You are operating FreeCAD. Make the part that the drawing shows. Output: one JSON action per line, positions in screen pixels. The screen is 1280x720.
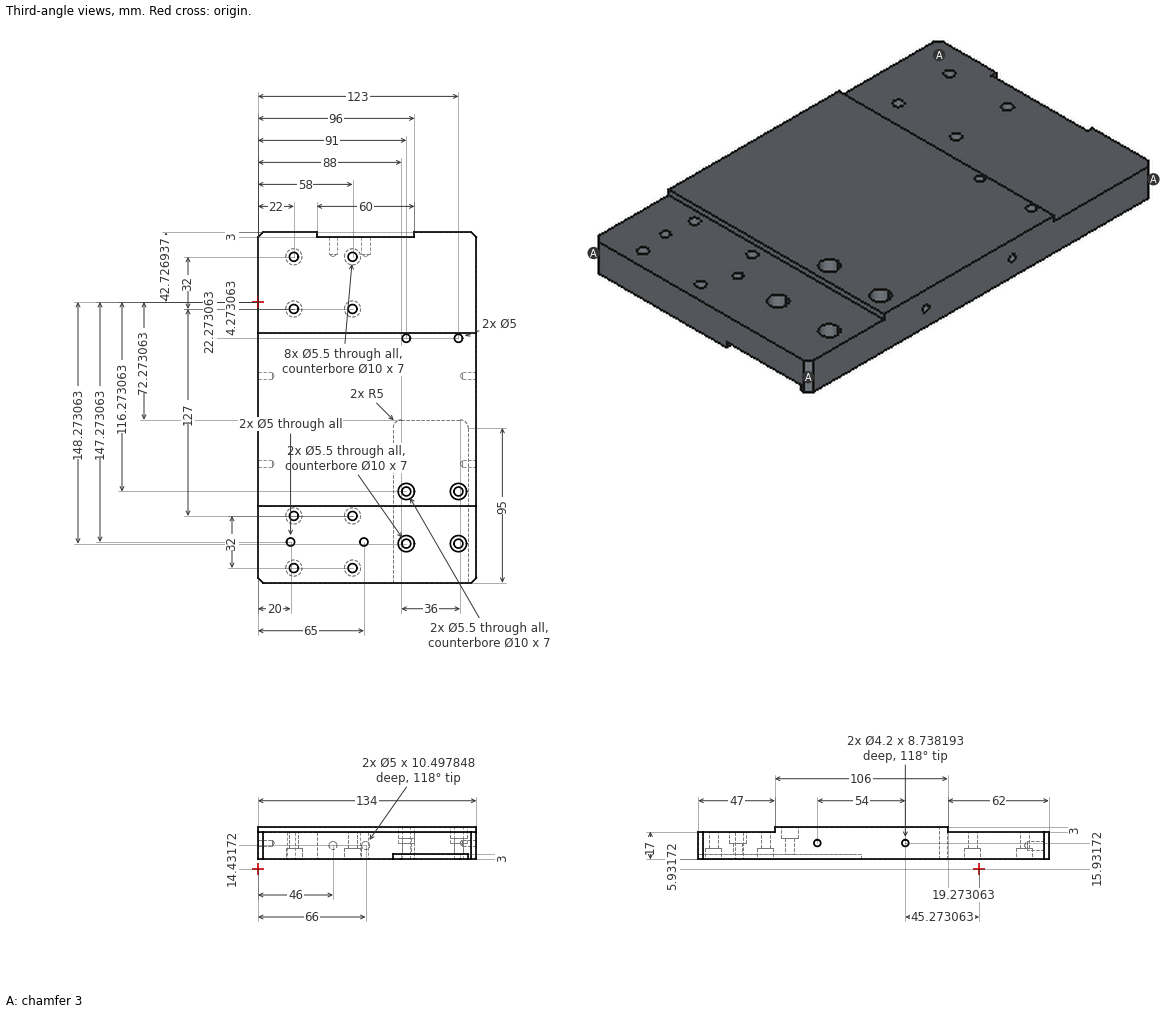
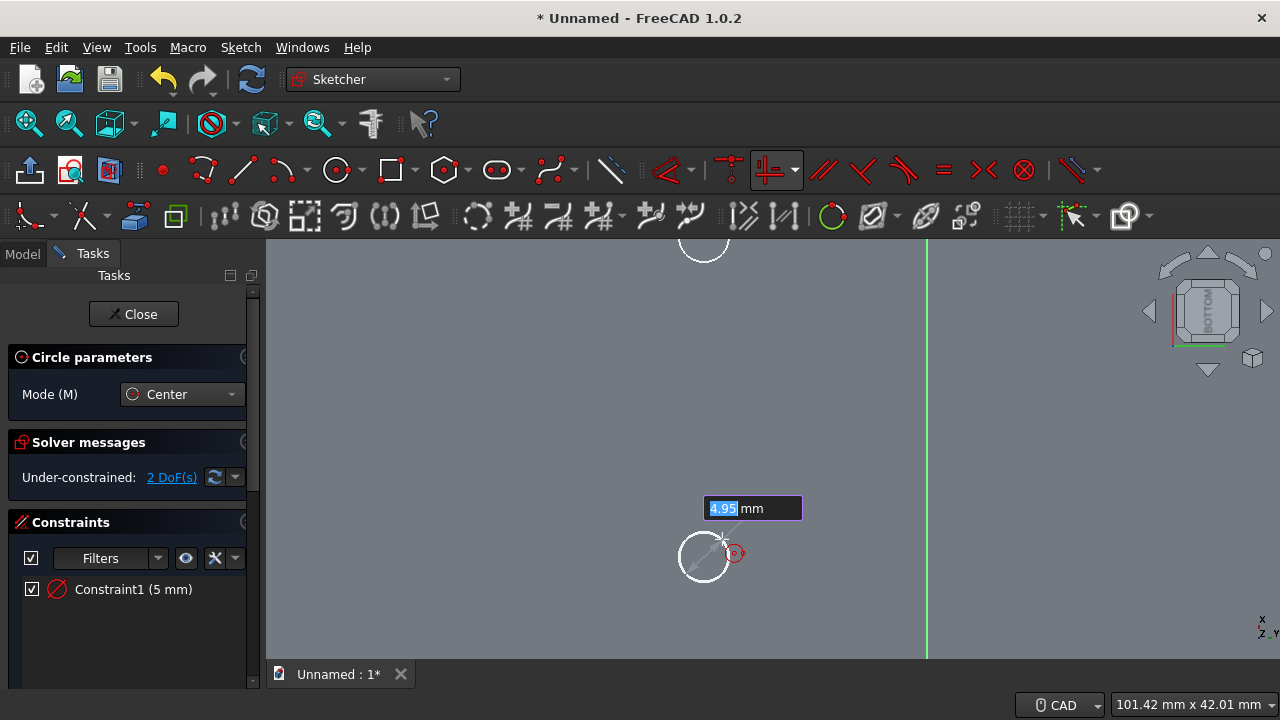
{"action": "type", "text": "5"}
{"action": "key", "text": "Return"}
{"action": "key", "text": "Escape"}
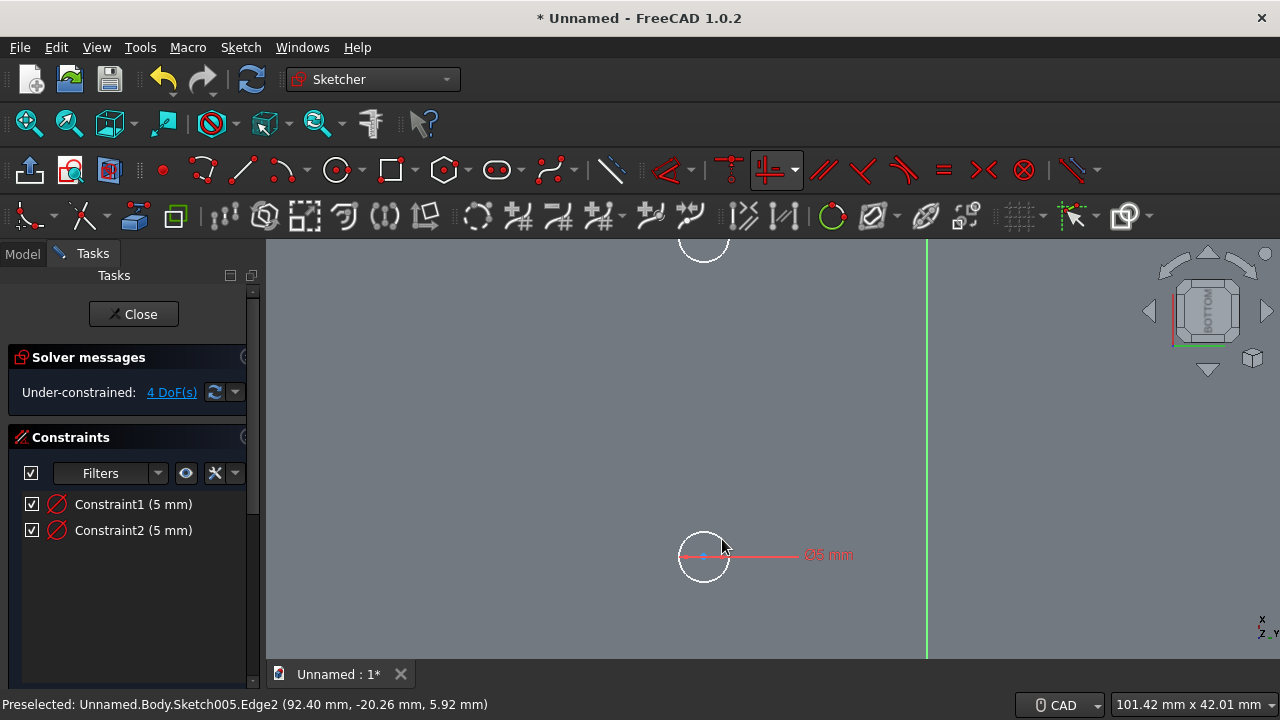
{"action": "scroll", "coordinate": [705, 556], "scroll_direction": "down", "scroll_amount": 2}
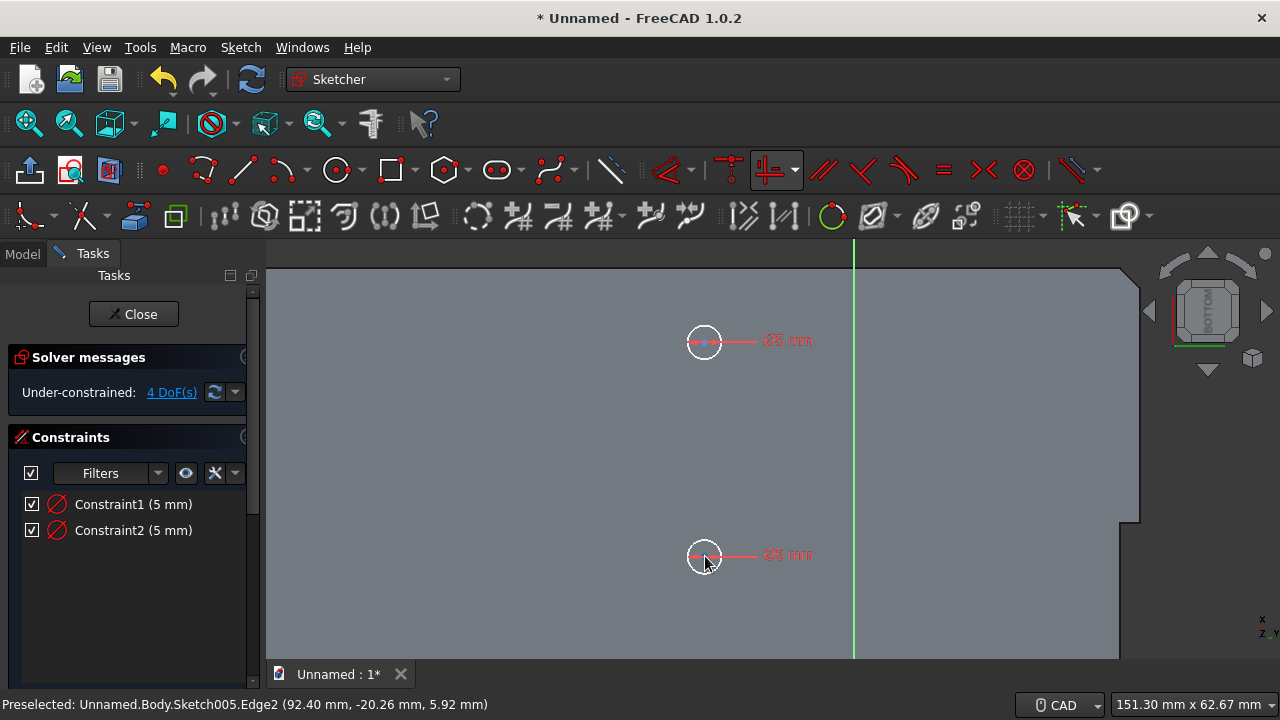
{"action": "left_click", "coordinate": [704, 342]}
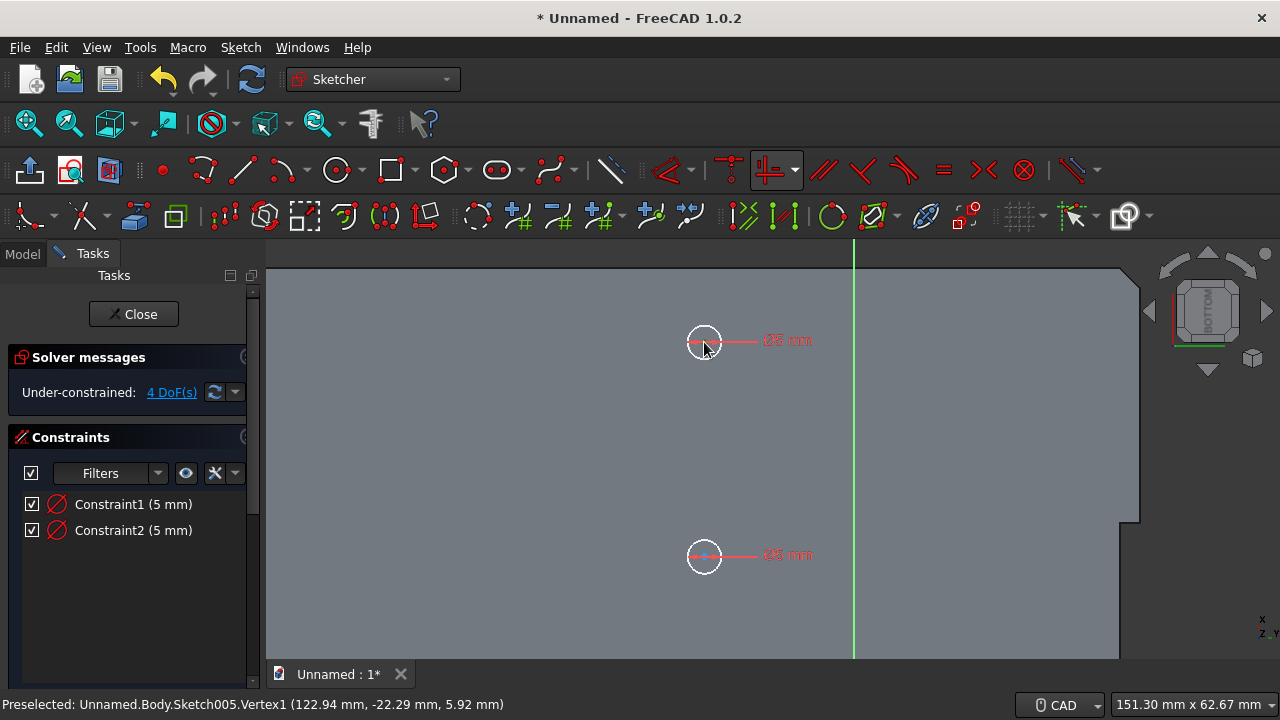
{"action": "left_click", "coordinate": [704, 557]}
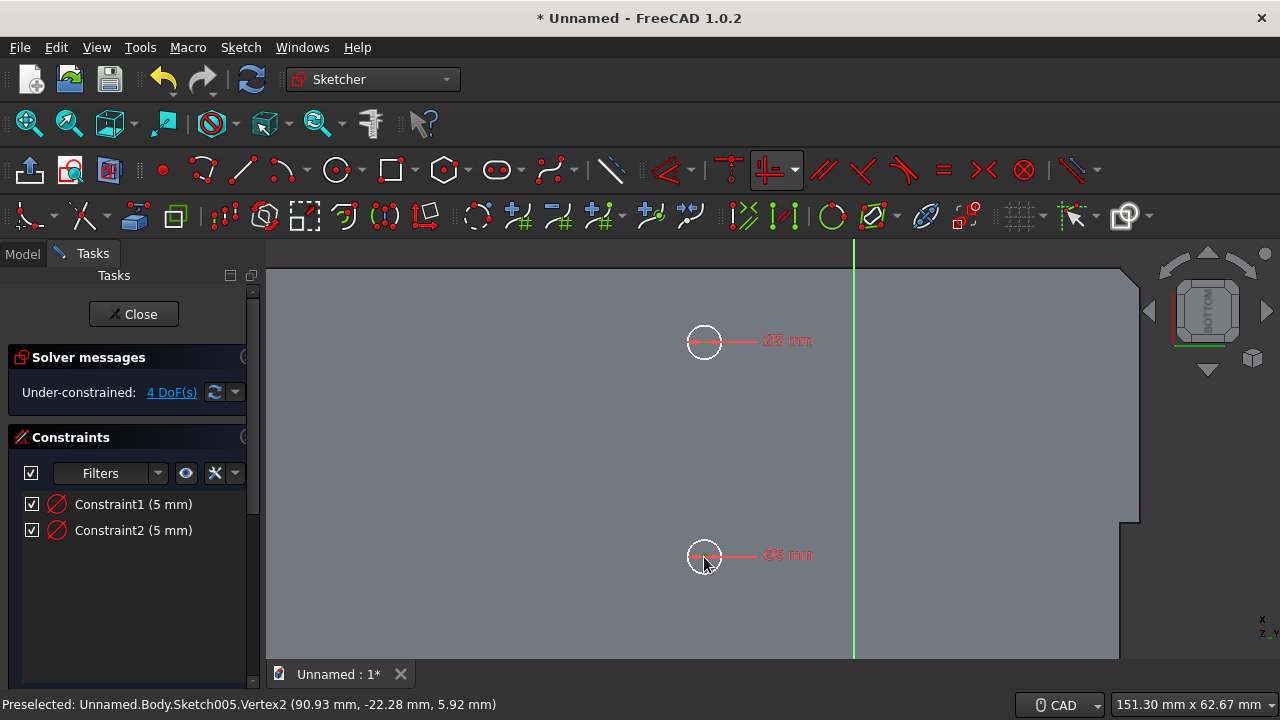
{"action": "key", "text": "v"}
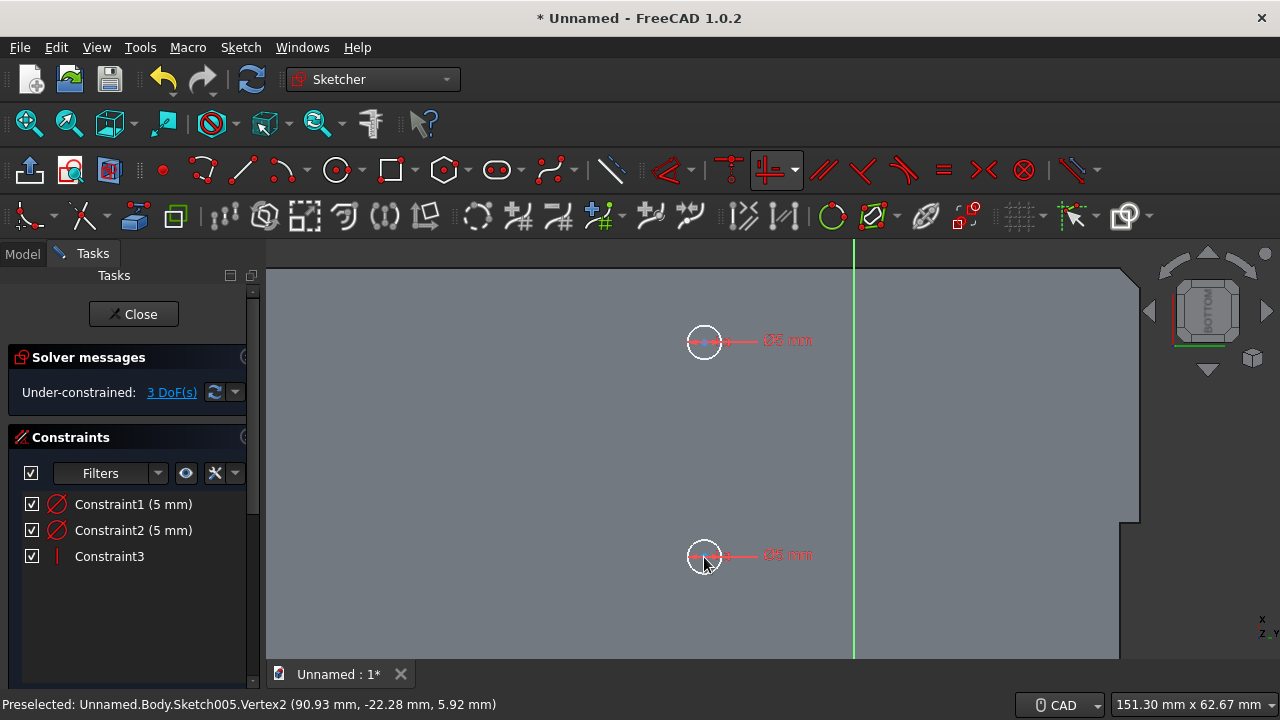
{"action": "left_click", "coordinate": [666, 170]}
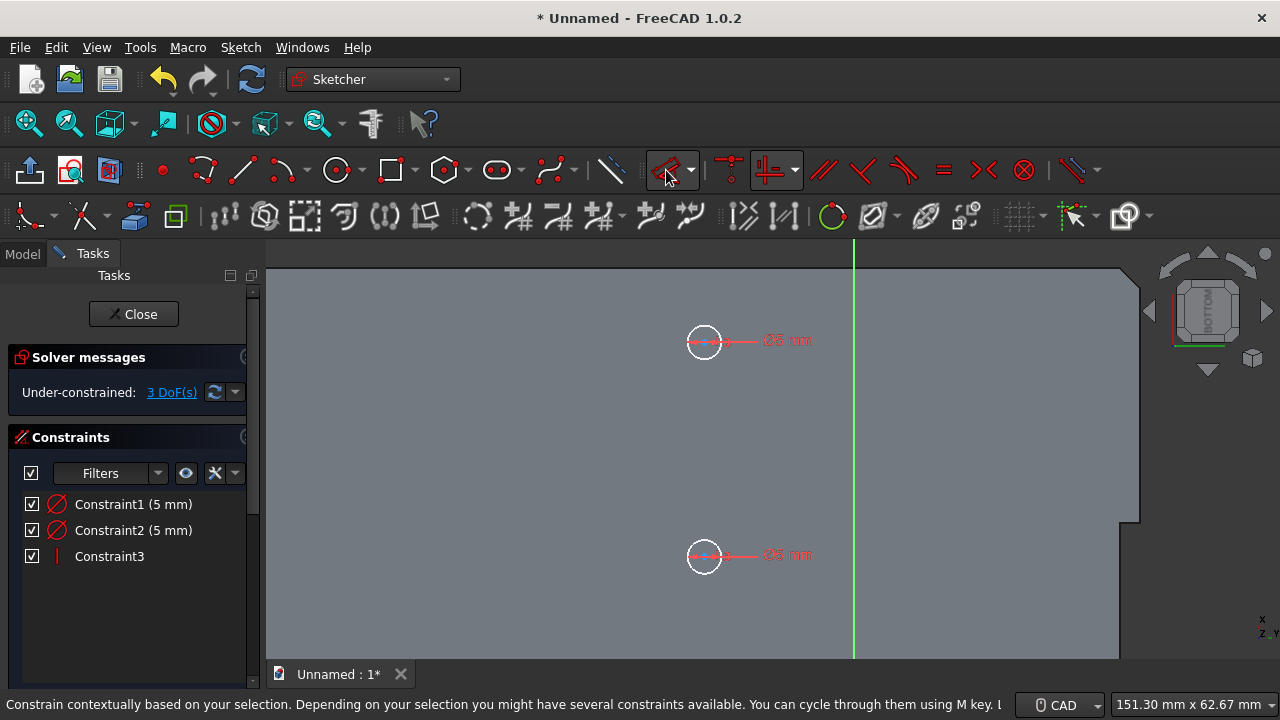
{"action": "left_click", "coordinate": [704, 557]}
{"action": "left_click", "coordinate": [888, 594]}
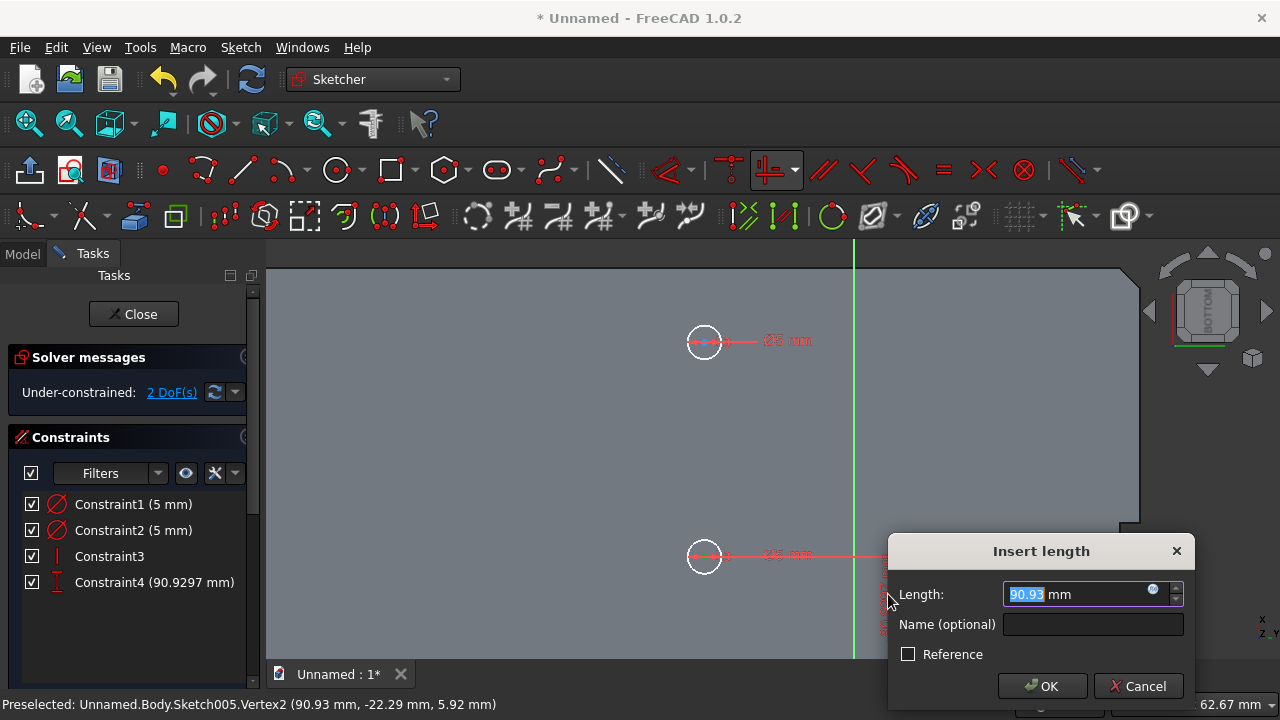
{"action": "type", "text": "91"}
{"action": "key", "text": "Return"}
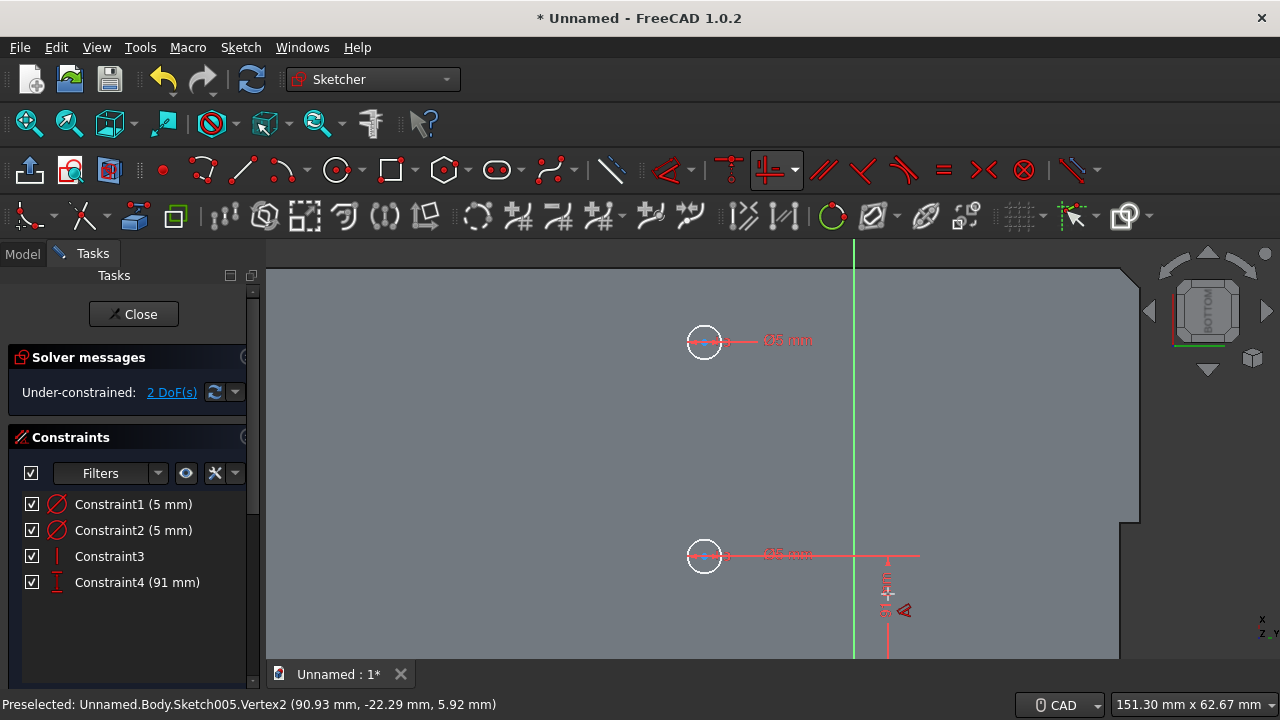
{"action": "left_click", "coordinate": [704, 342]}
{"action": "left_click", "coordinate": [888, 487]}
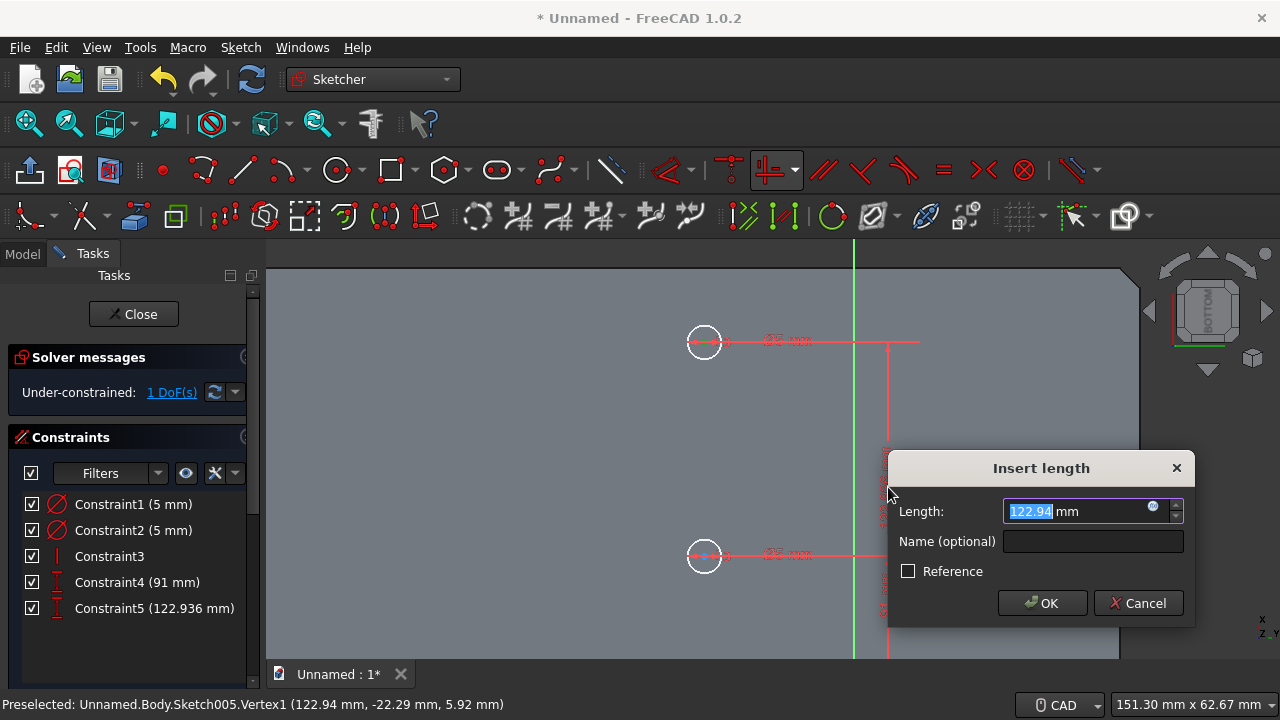
{"action": "type", "text": "123"}
{"action": "key", "text": "Return"}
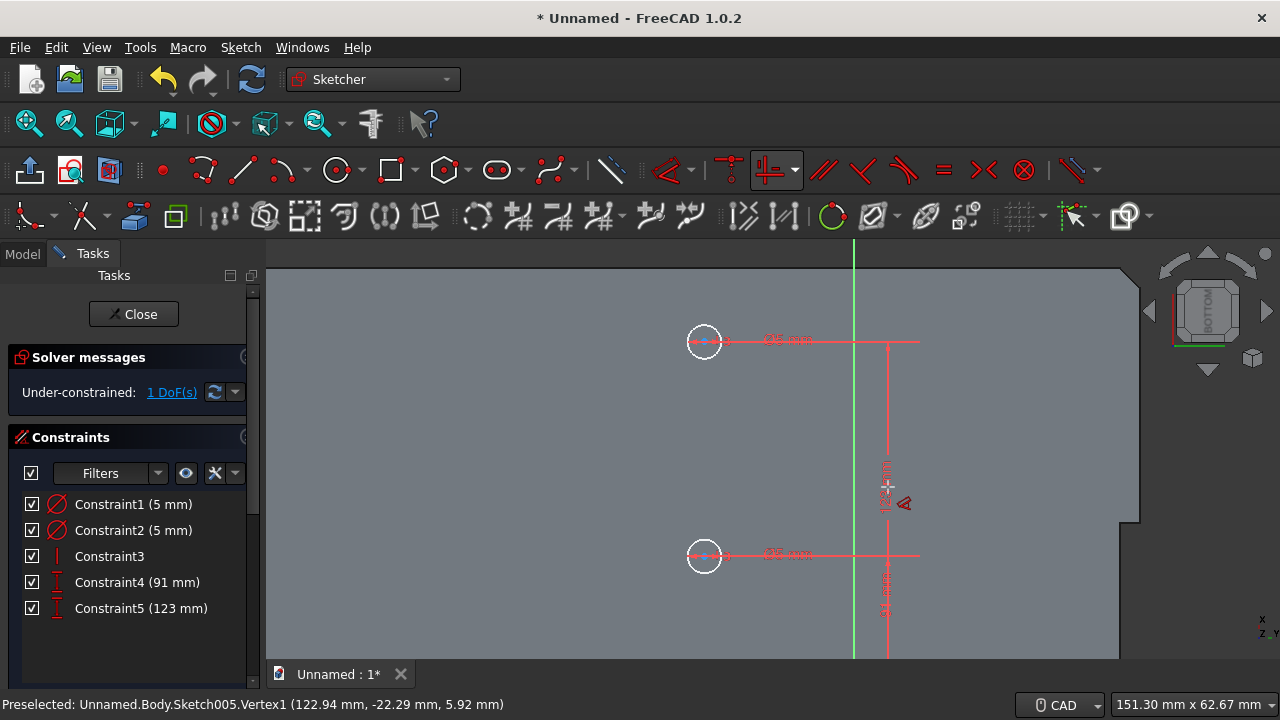
{"action": "left_click", "coordinate": [704, 342]}
{"action": "left_click", "coordinate": [779, 308]}